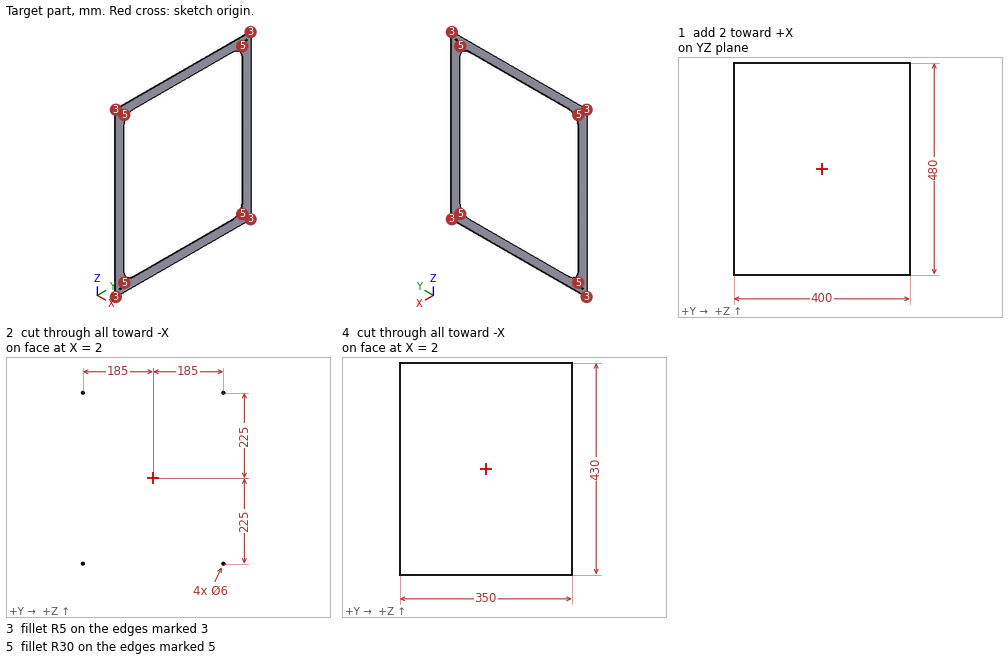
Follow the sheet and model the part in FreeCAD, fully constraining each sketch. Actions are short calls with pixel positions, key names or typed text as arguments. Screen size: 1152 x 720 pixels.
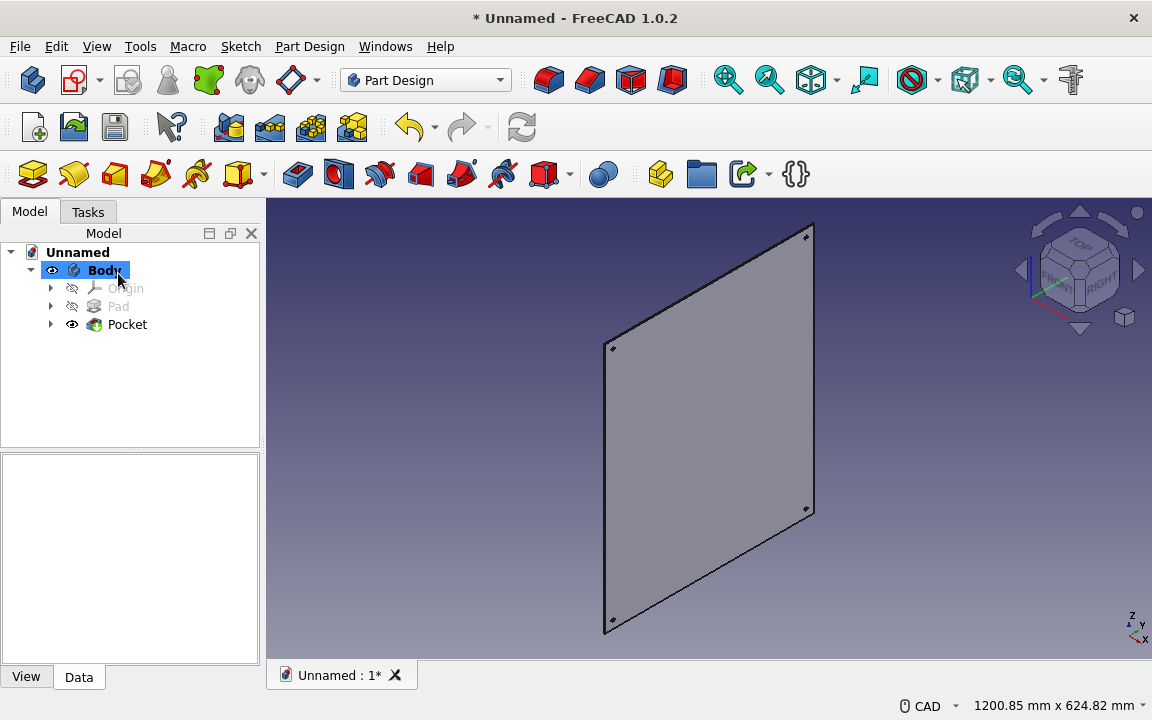
key(2)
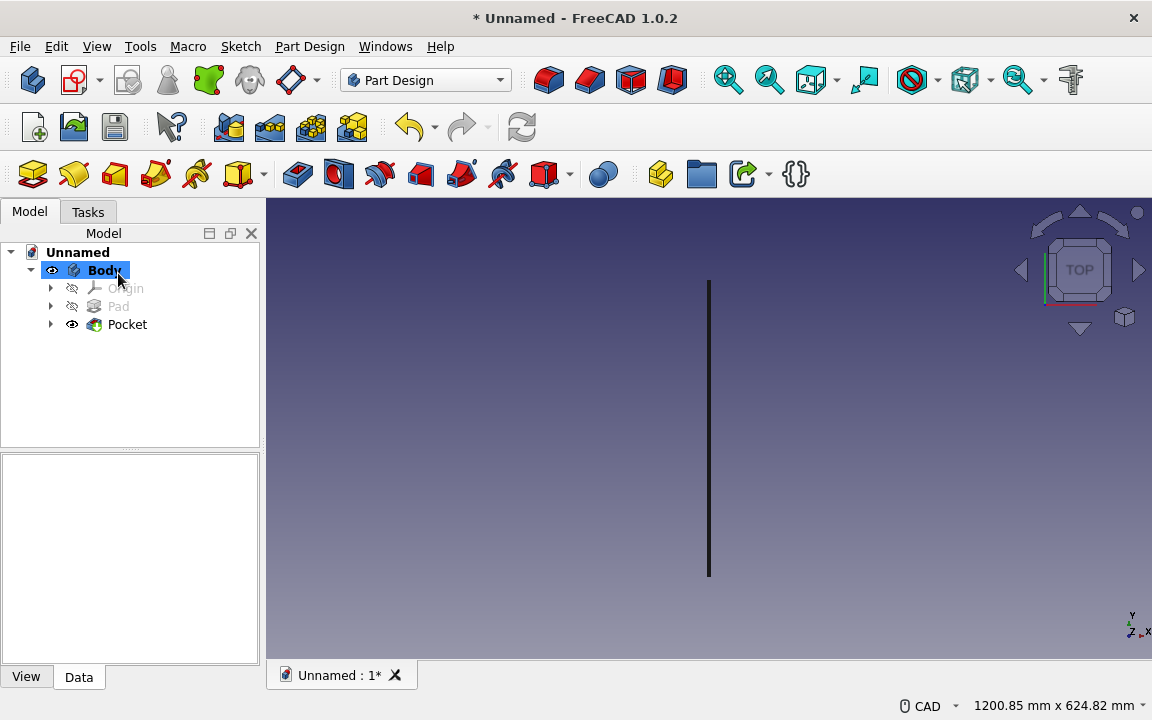
scroll(709, 280, up, 15)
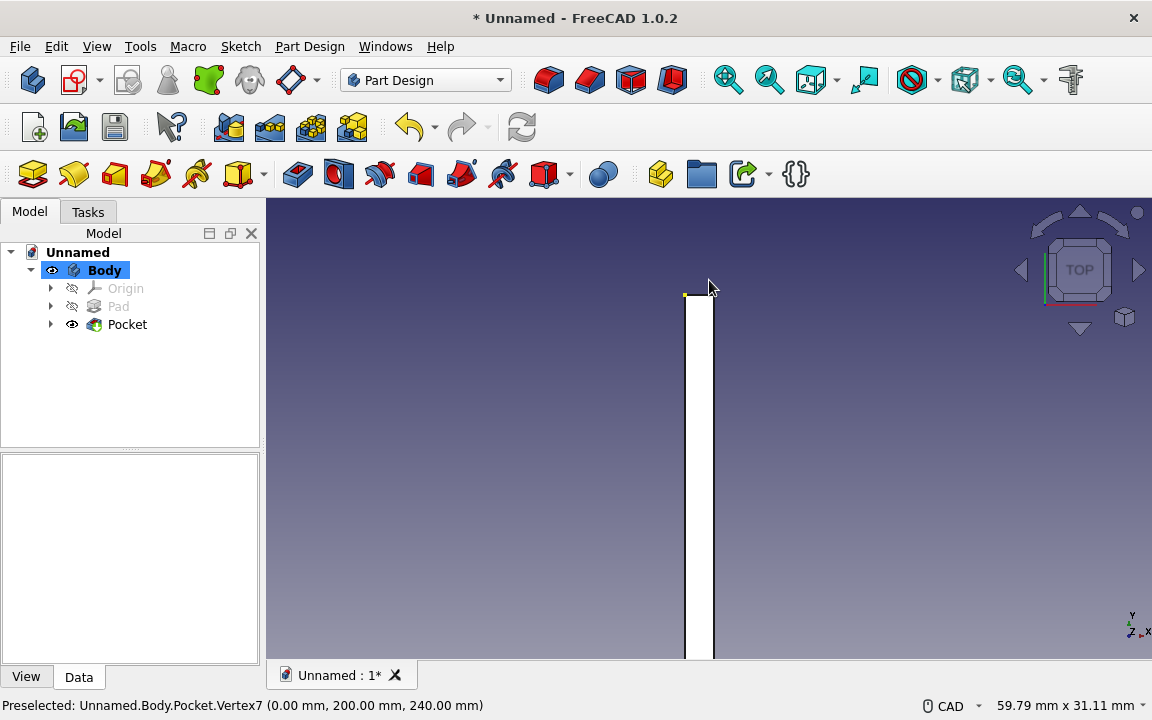
click(699, 294)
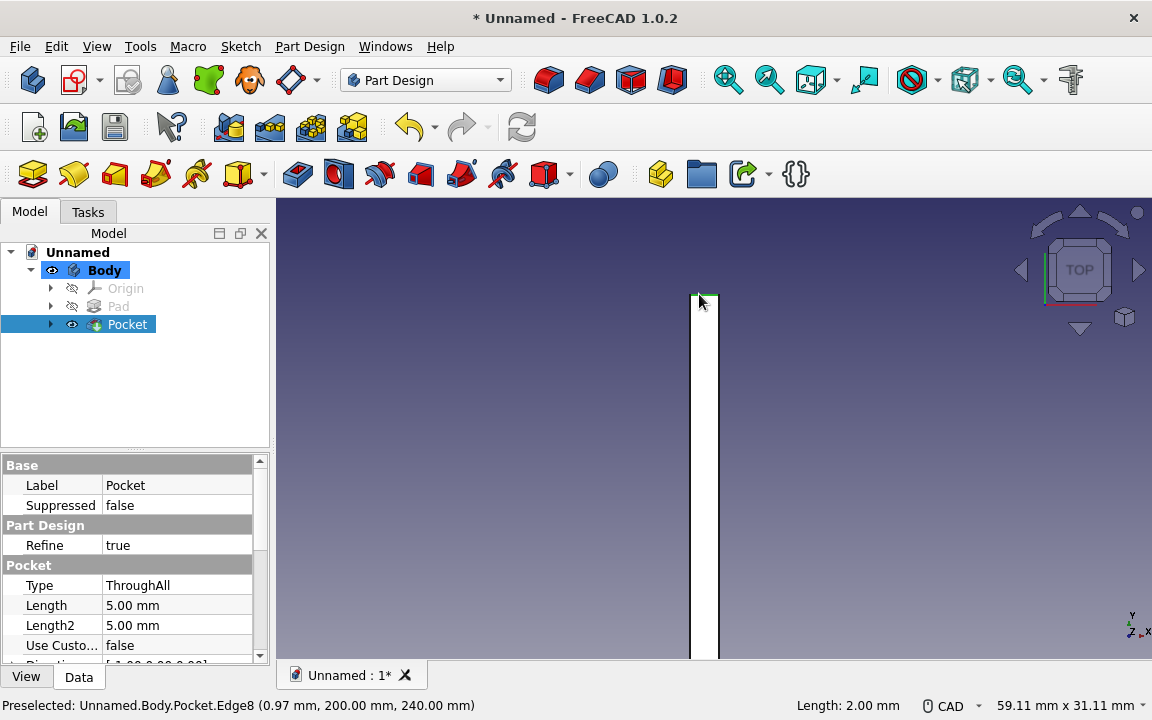
key(v)
key(f)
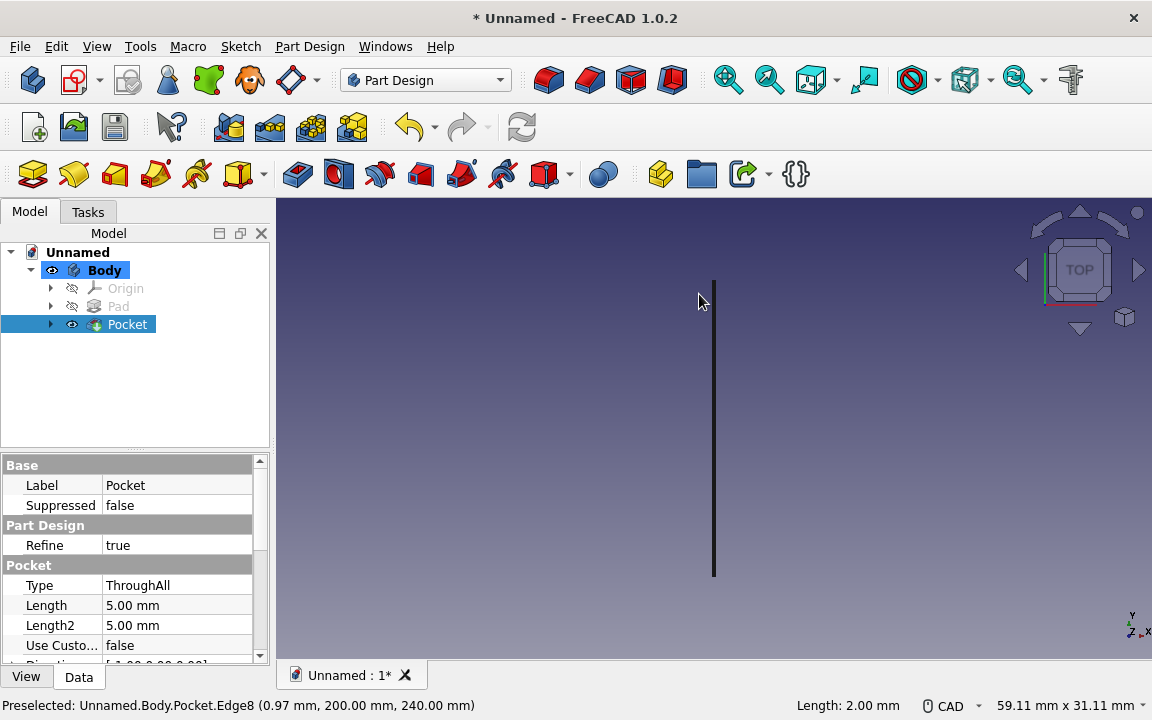
key(1)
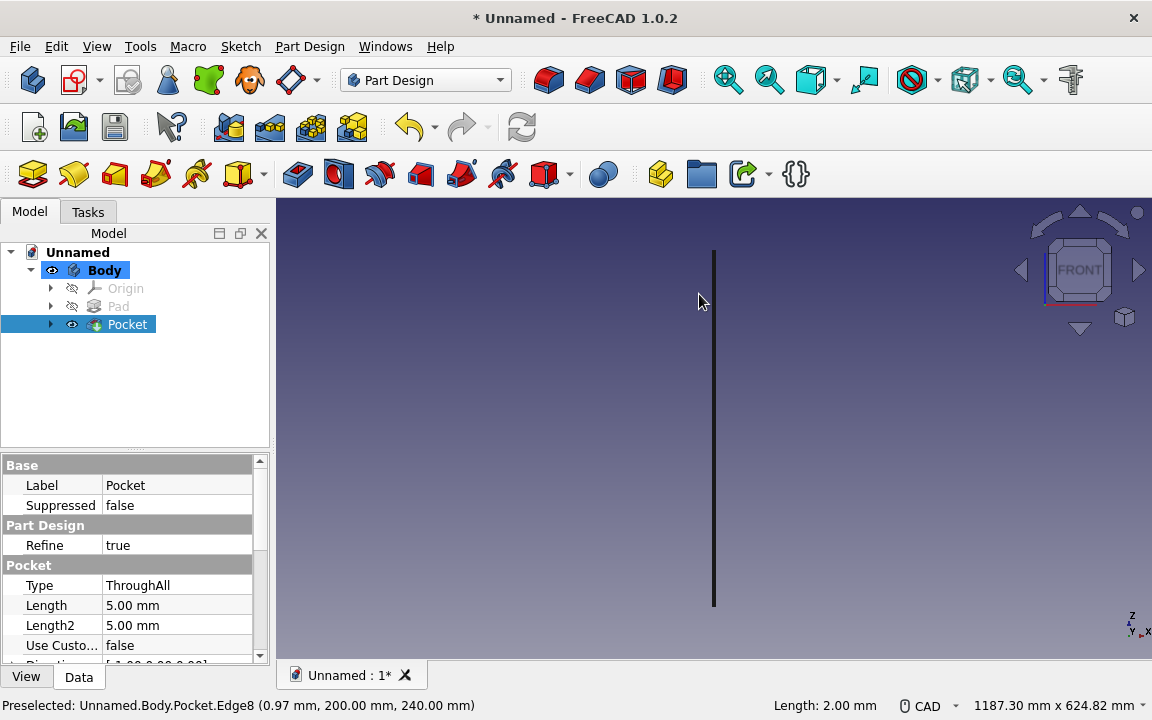
scroll(714, 605, up, 15)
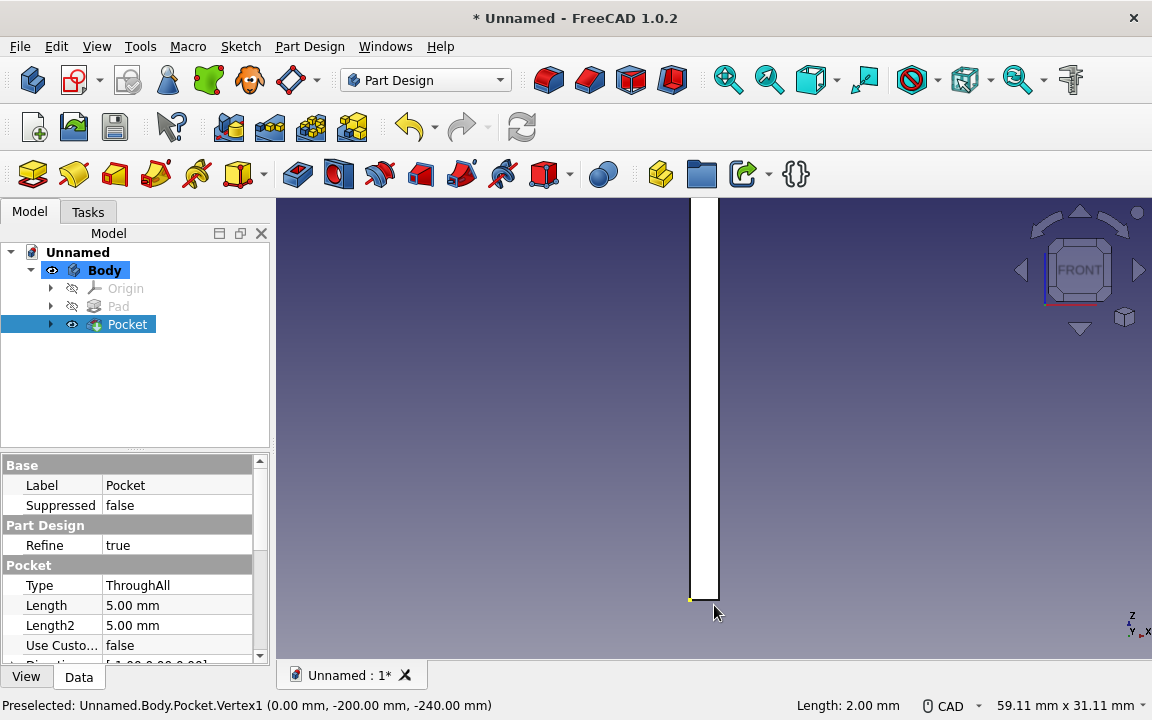
click(704, 599, ctrl)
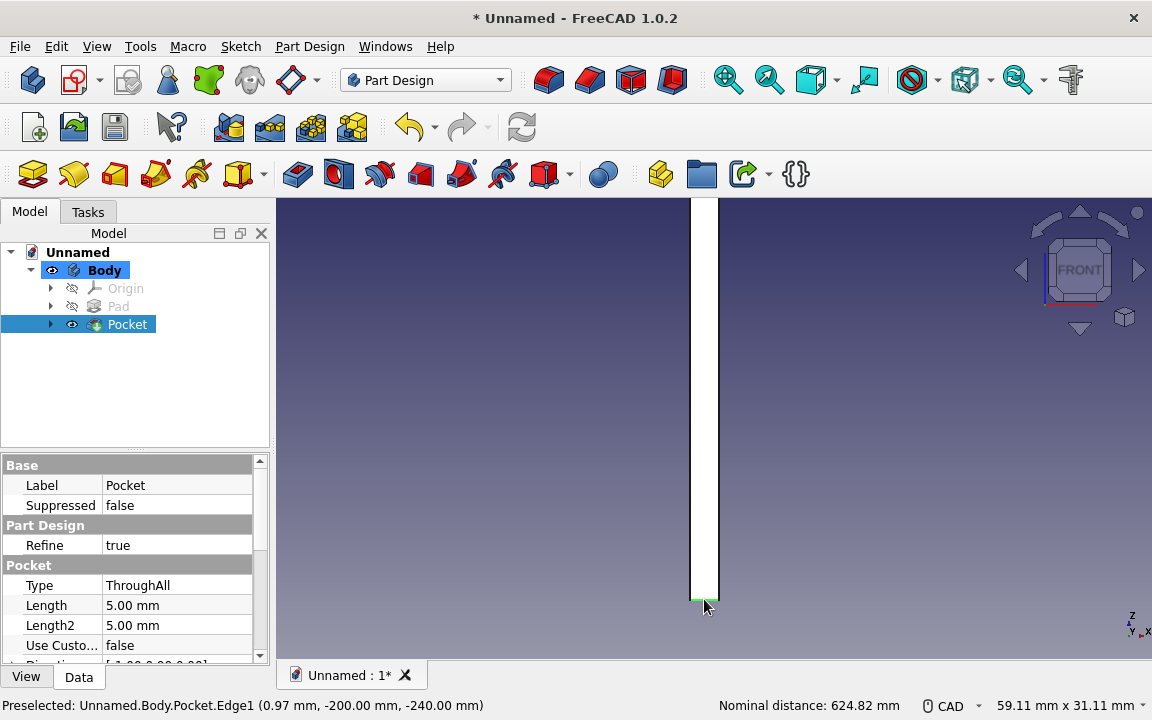
key(v)
key(f)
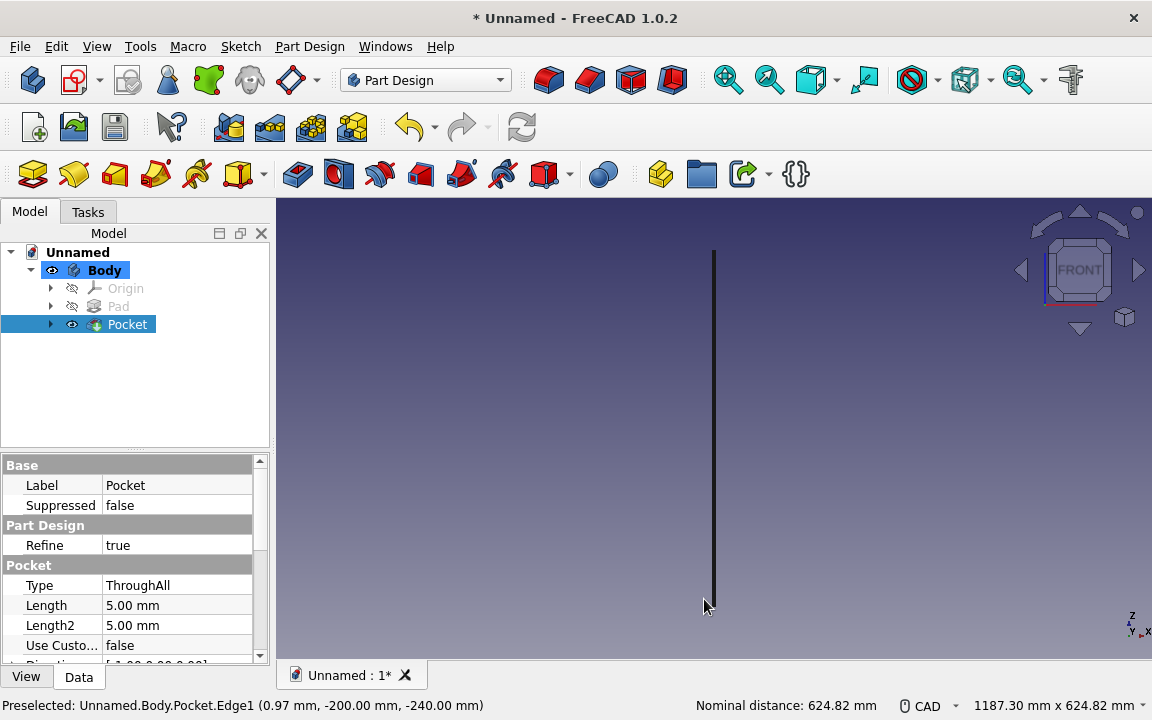
key(3)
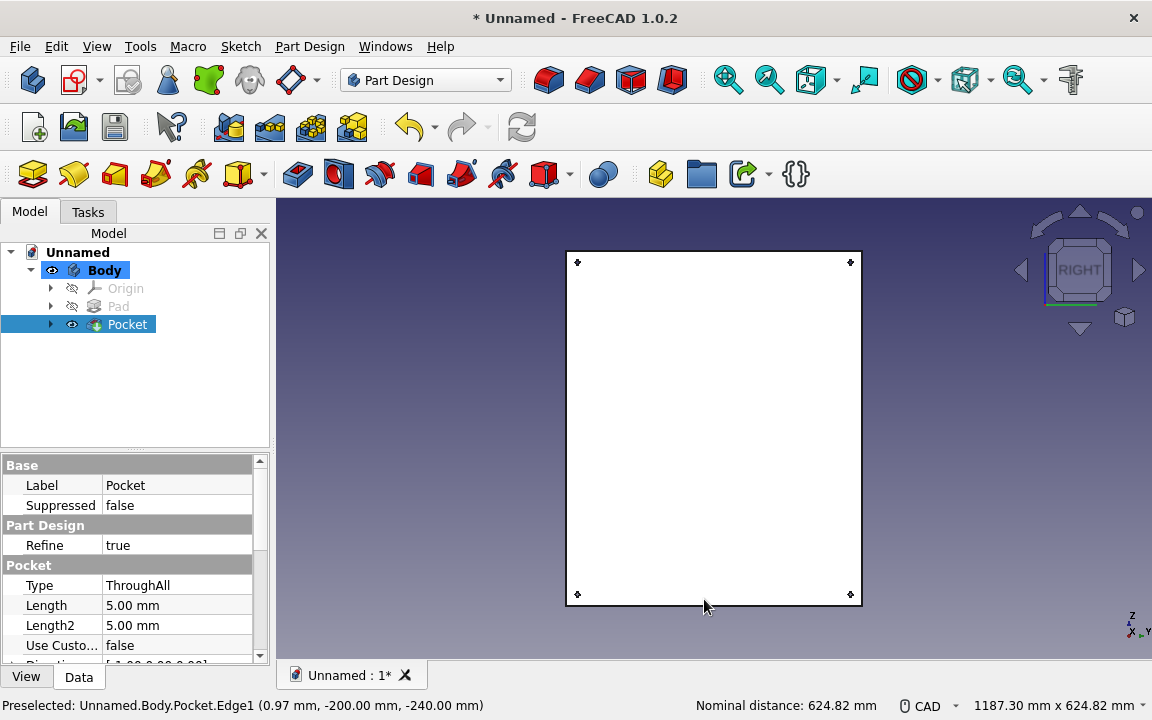
scroll(862, 605, up, 15)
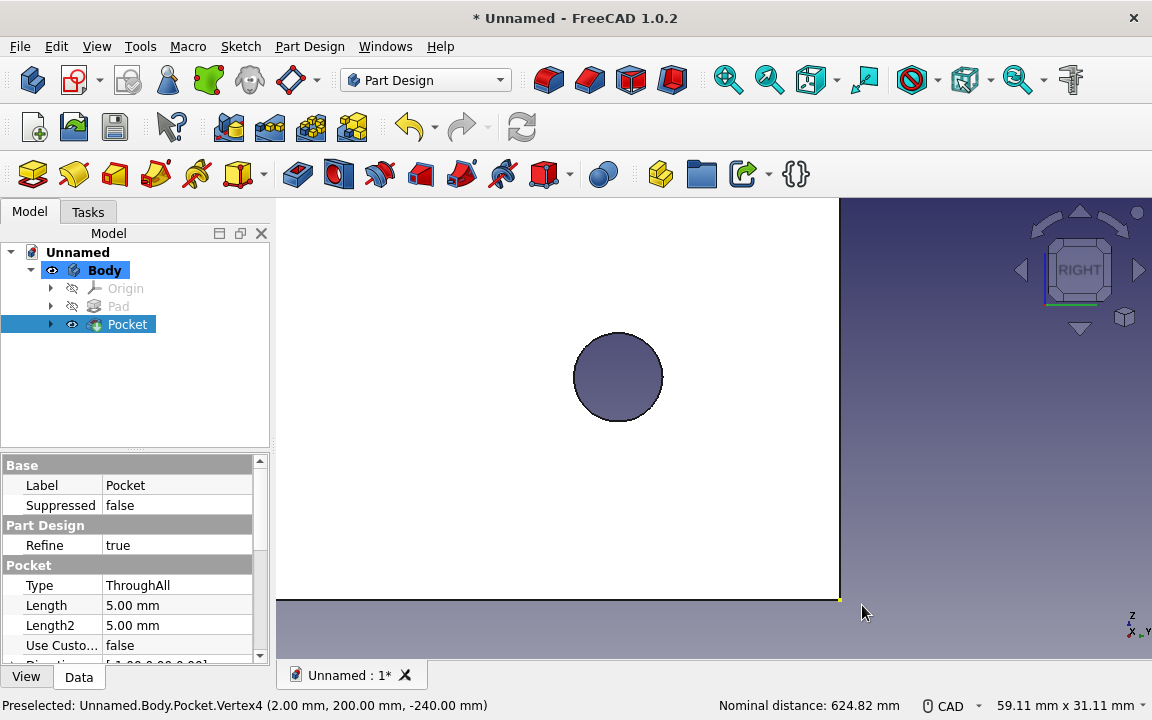
click(729, 80)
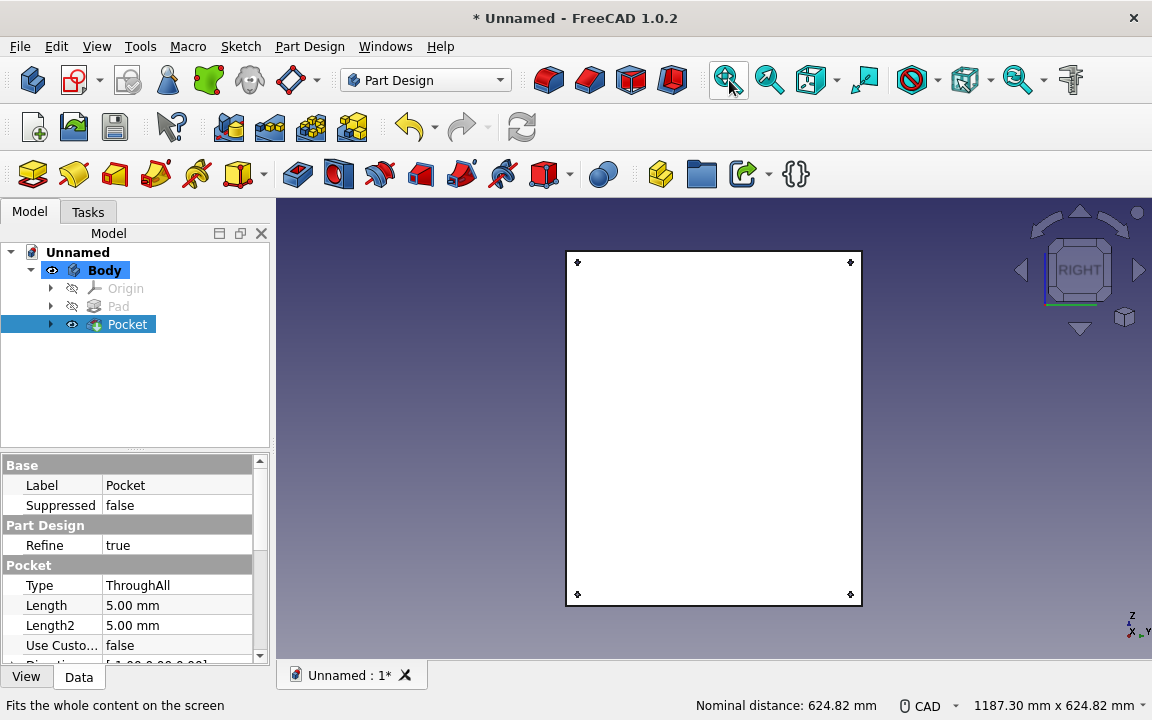
key(5)